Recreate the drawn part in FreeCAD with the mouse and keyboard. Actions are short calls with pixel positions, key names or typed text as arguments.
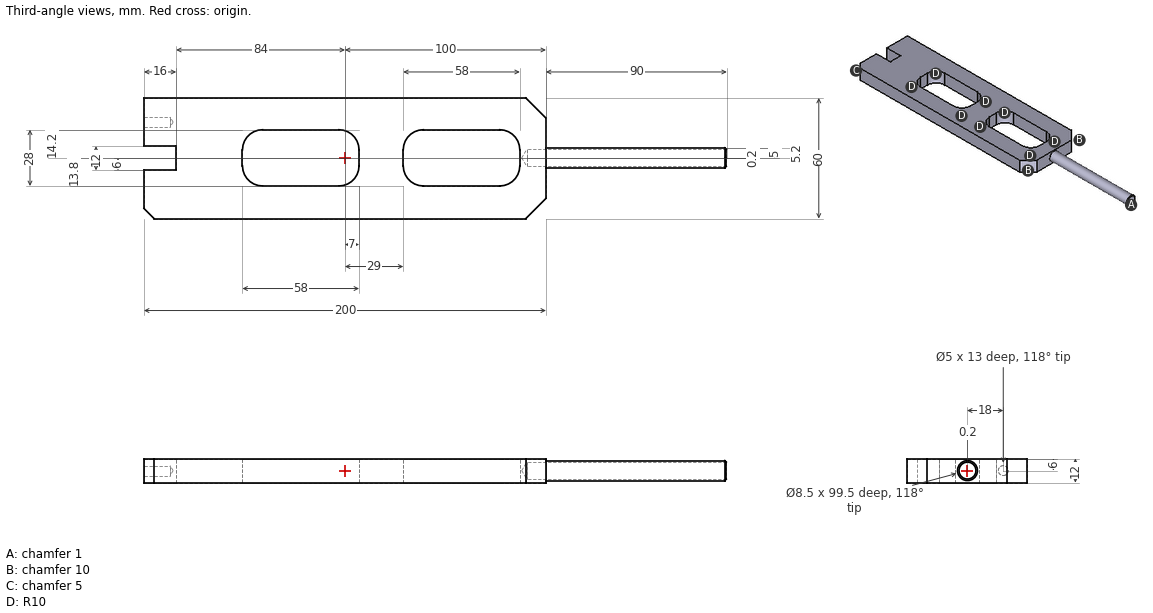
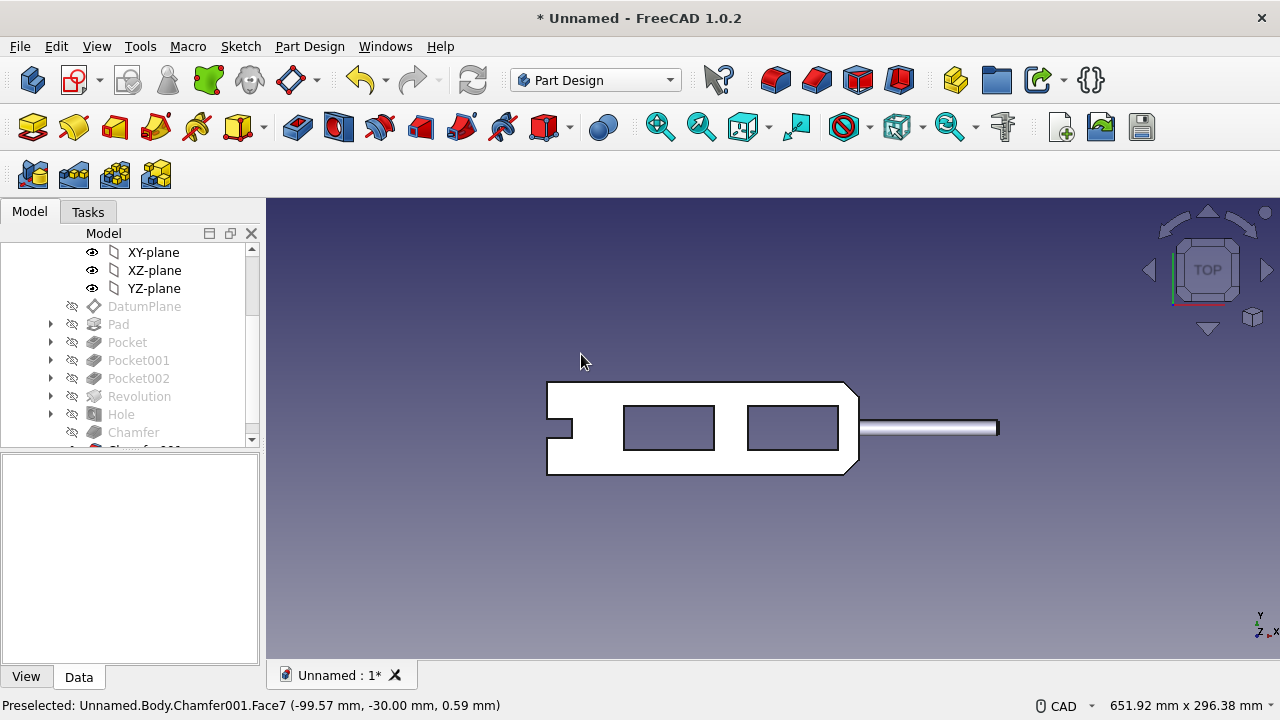
scroll(547, 474, up, 4)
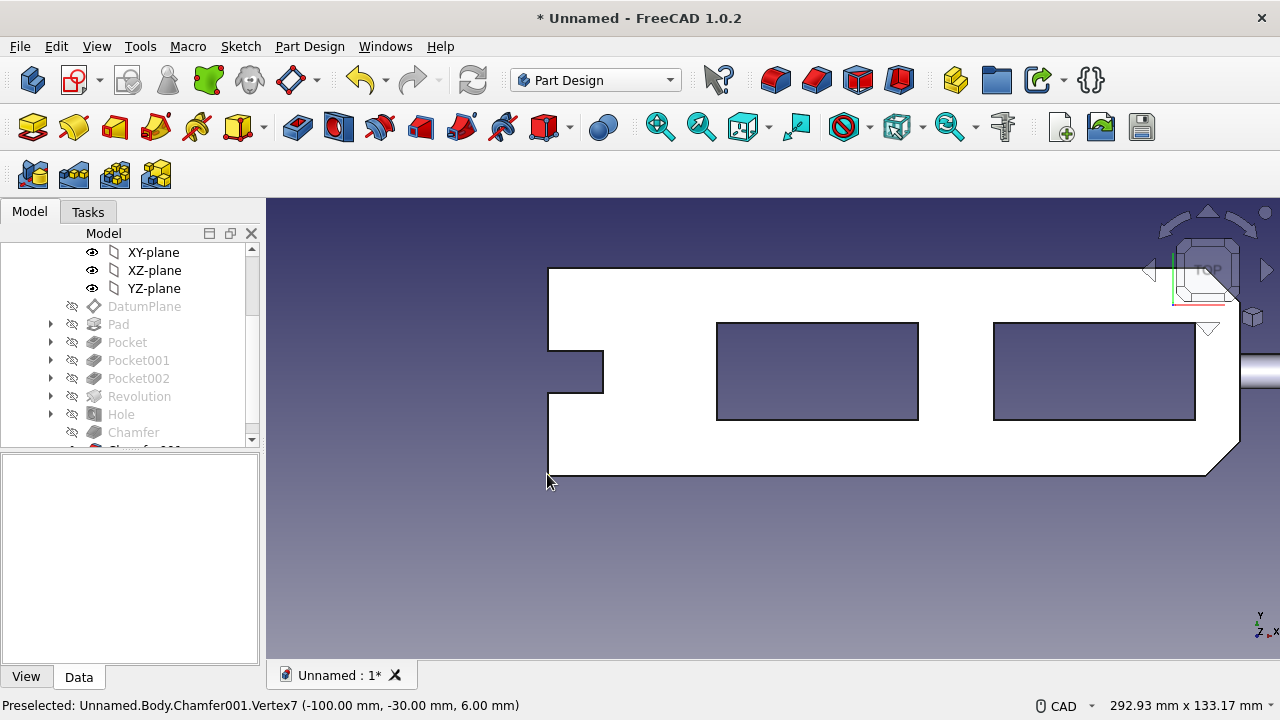
key(v)
key(f)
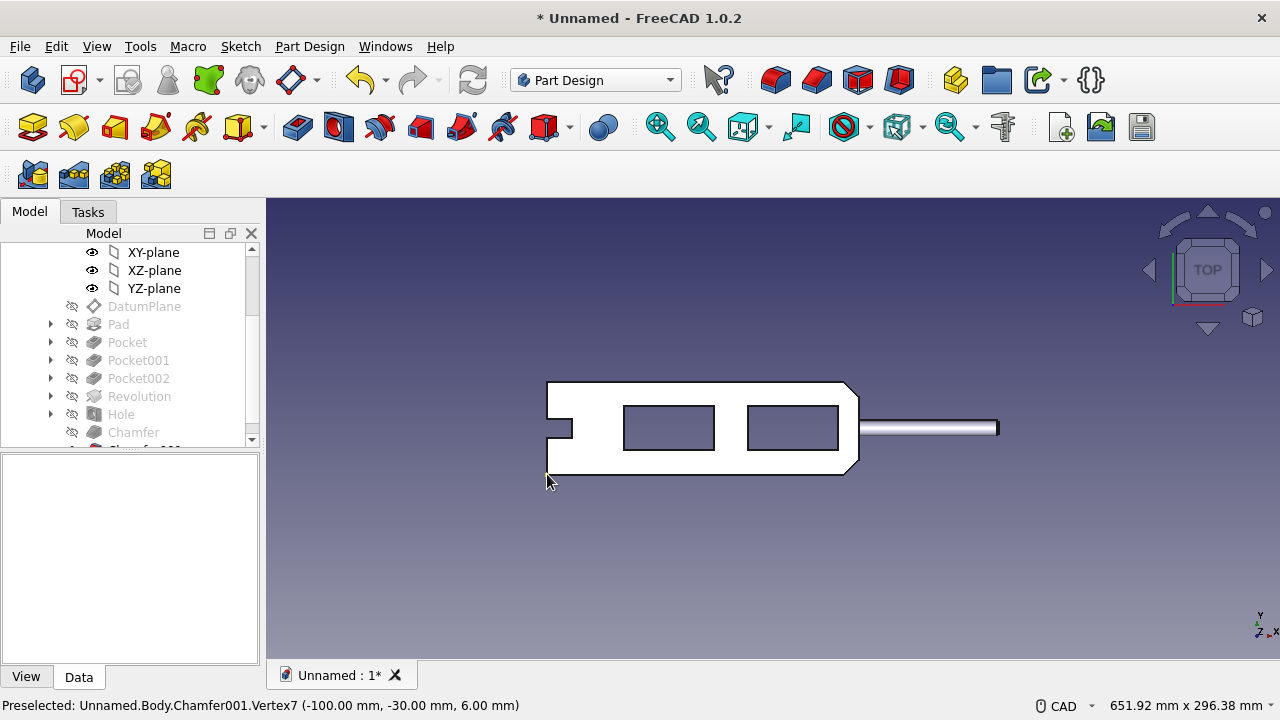
key(1)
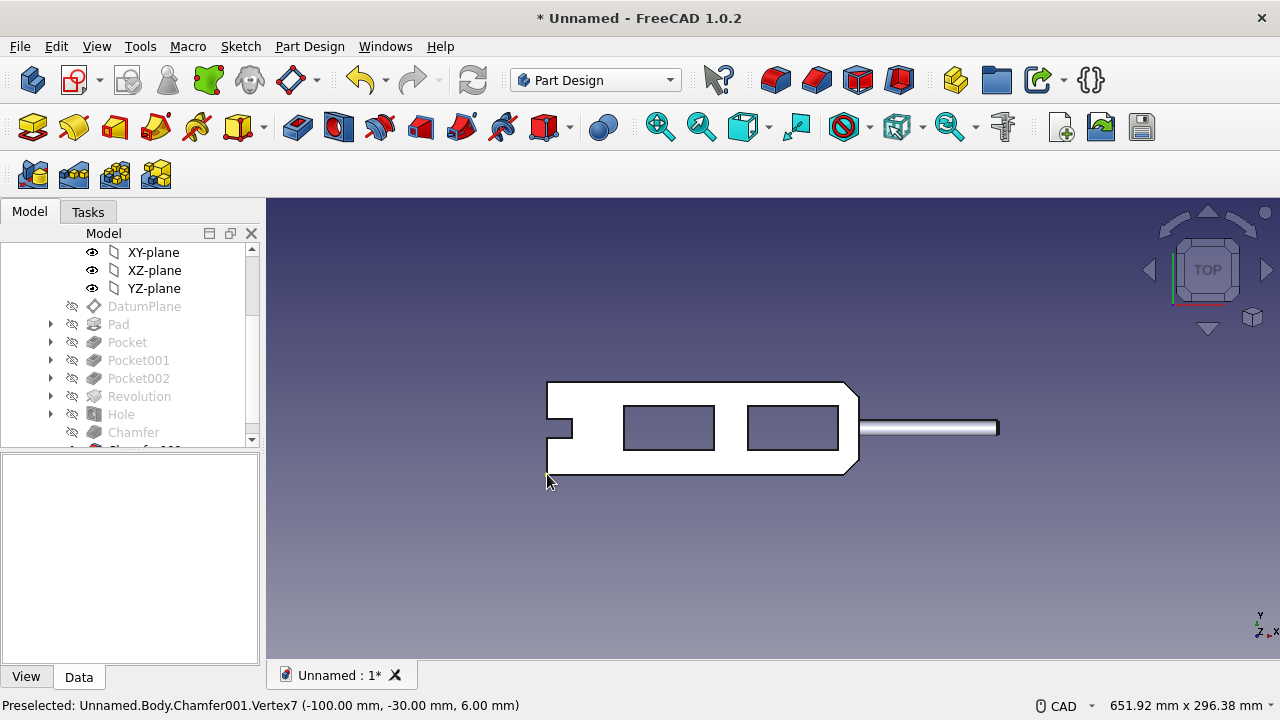
click(661, 128)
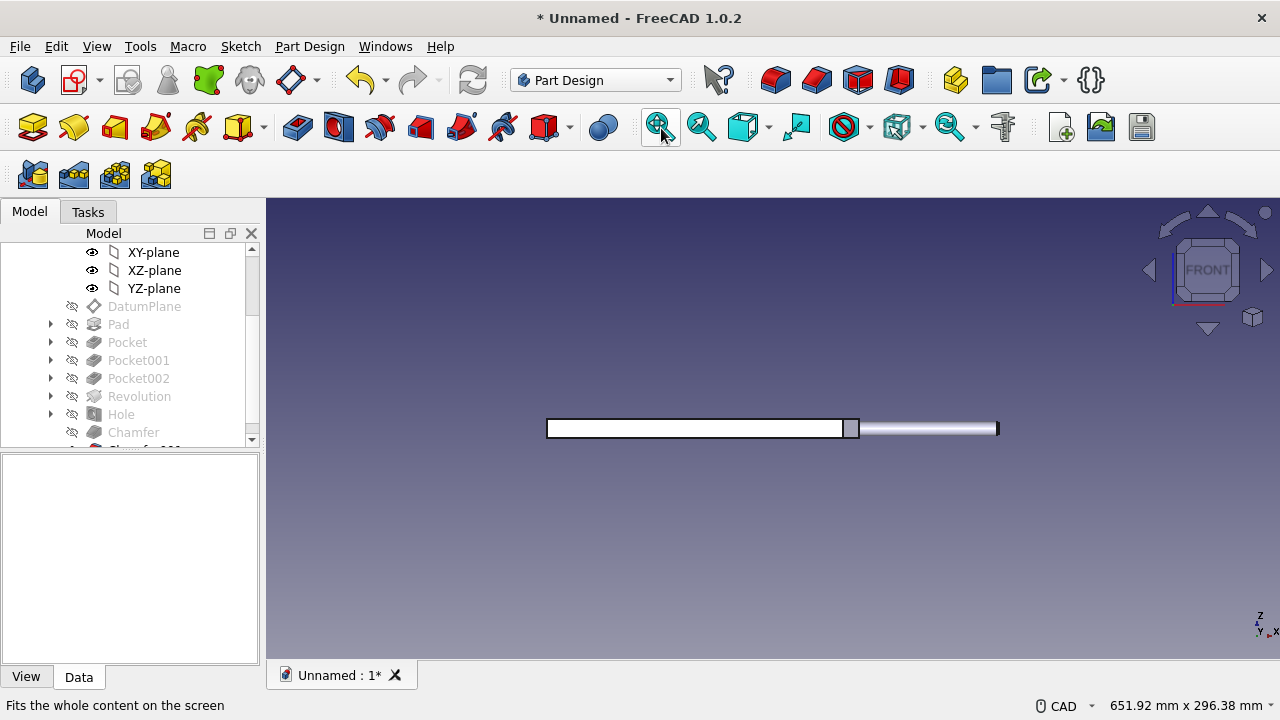
click(547, 428)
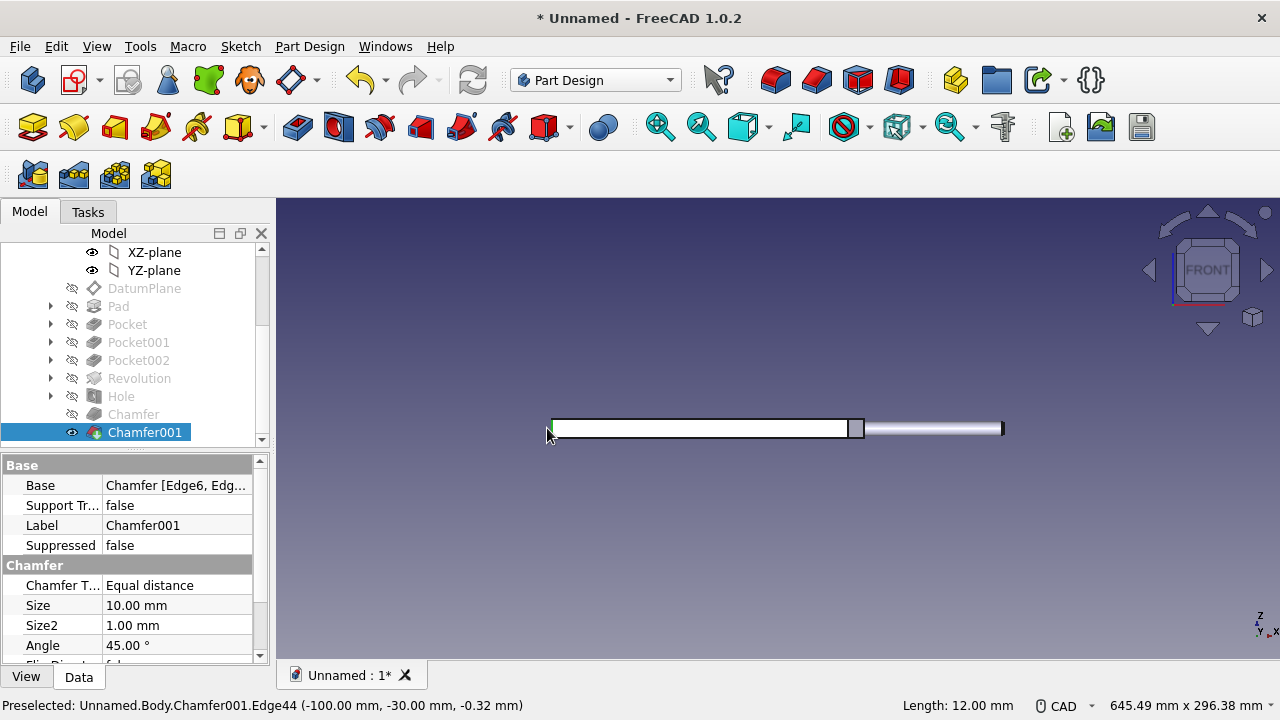
click(817, 80)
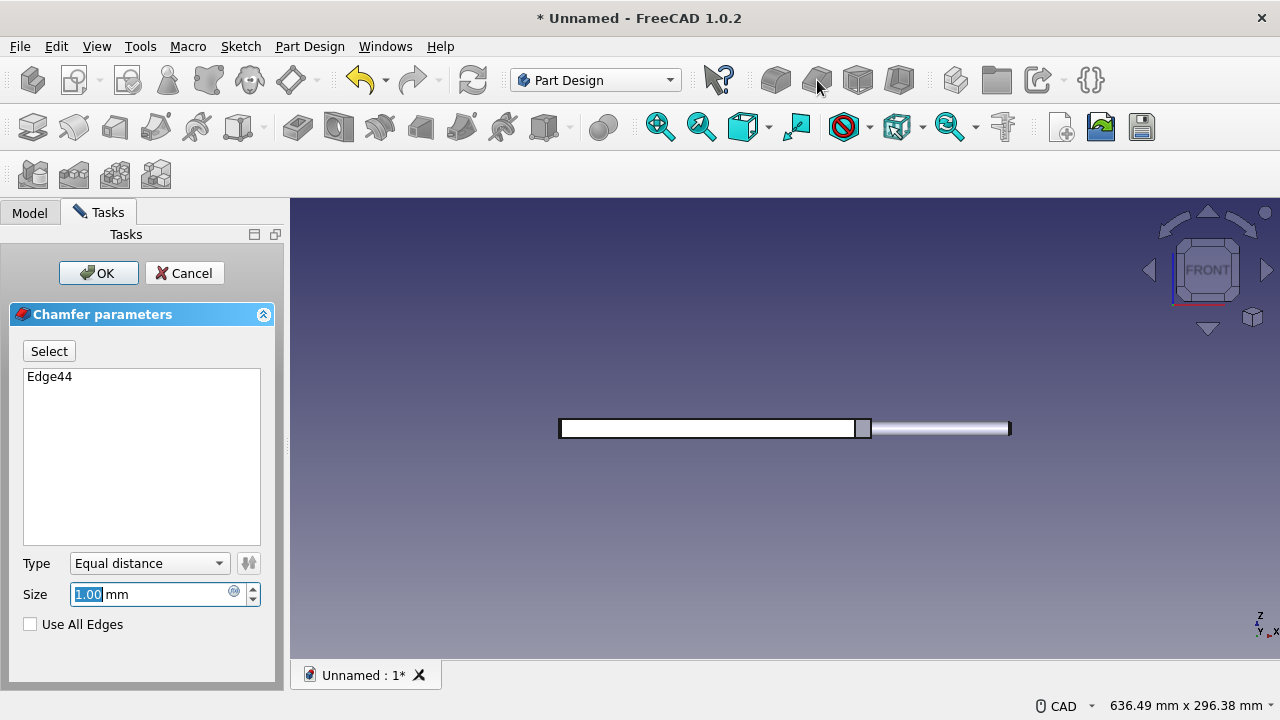
text(5)
key(Tab)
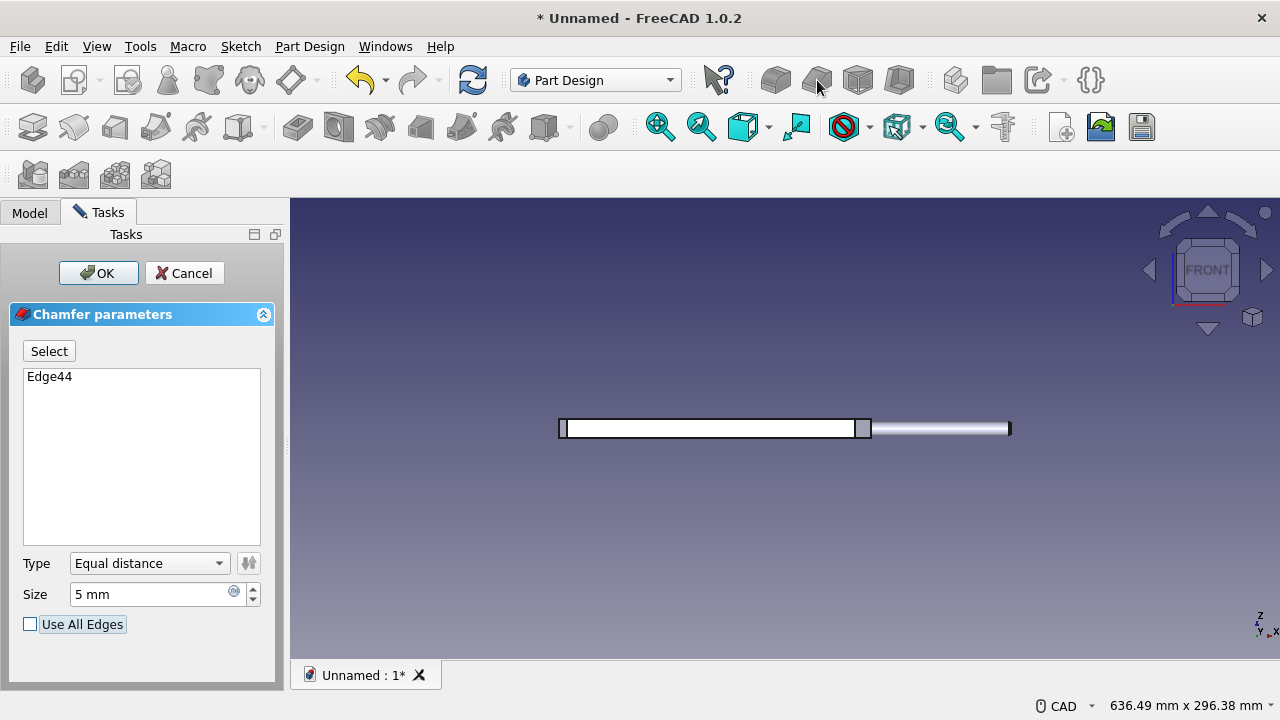
click(99, 273)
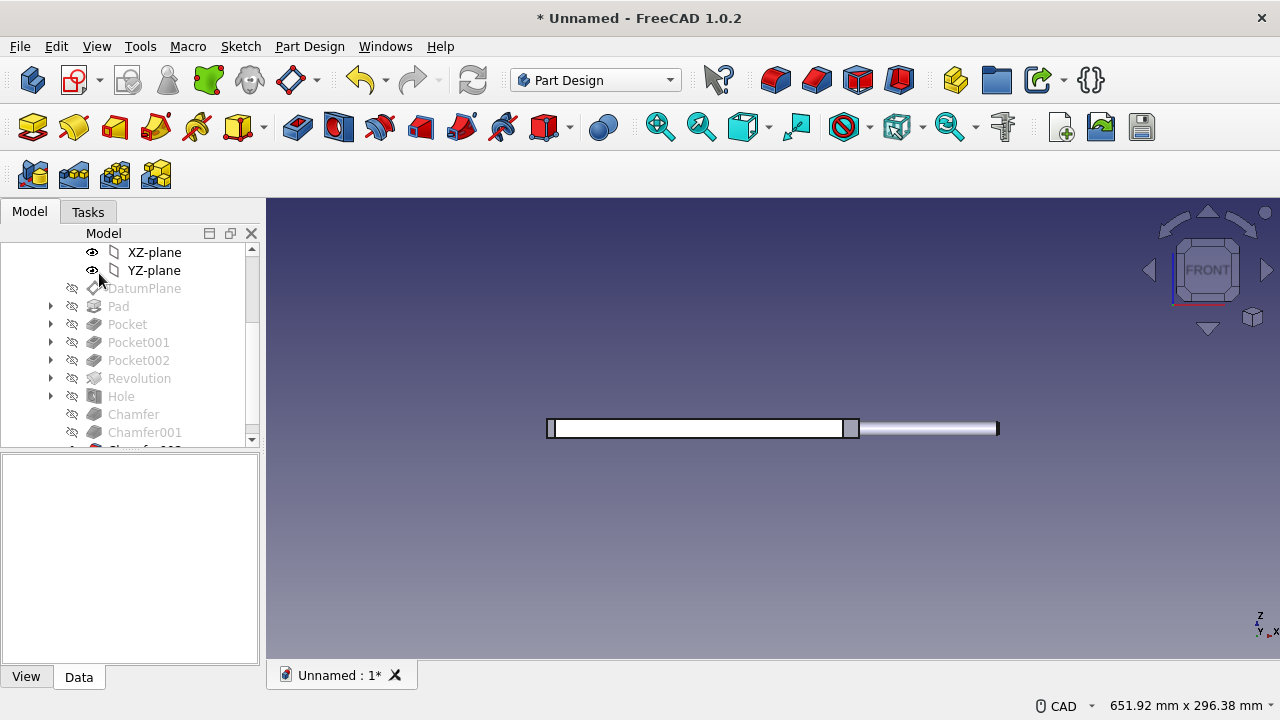
key(v)
key(f)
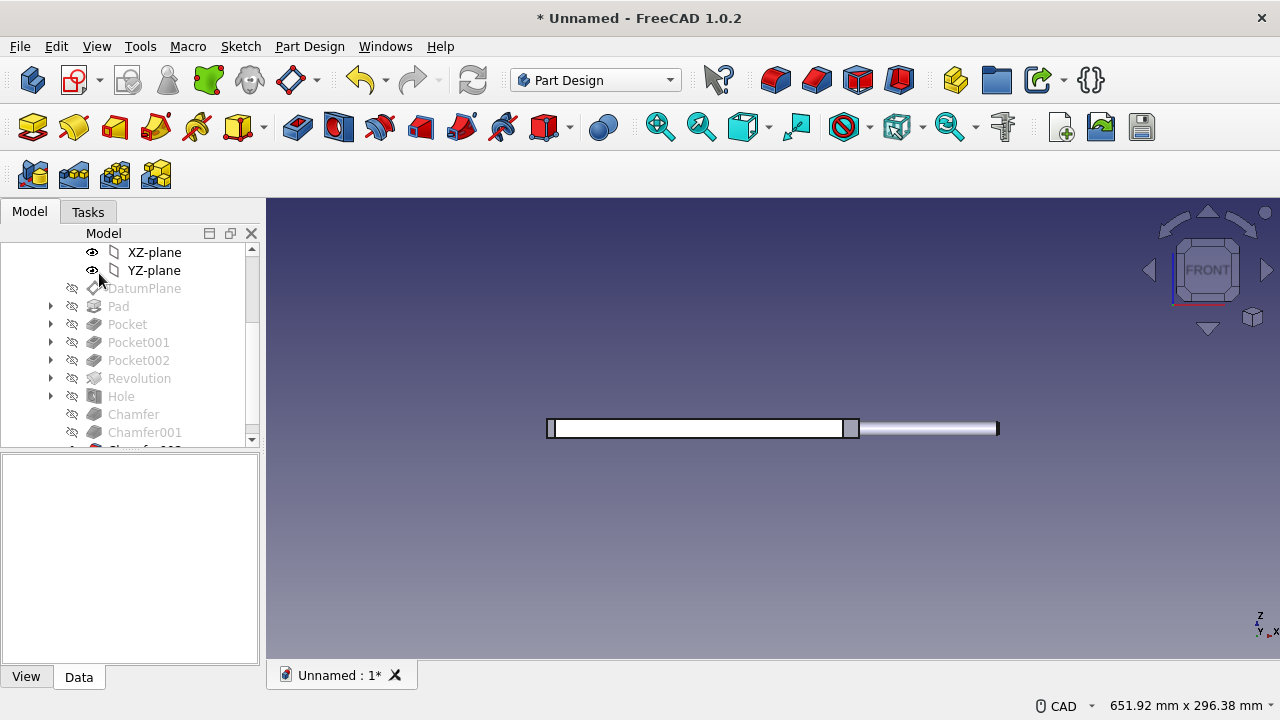
scroll(624, 428, up, 4)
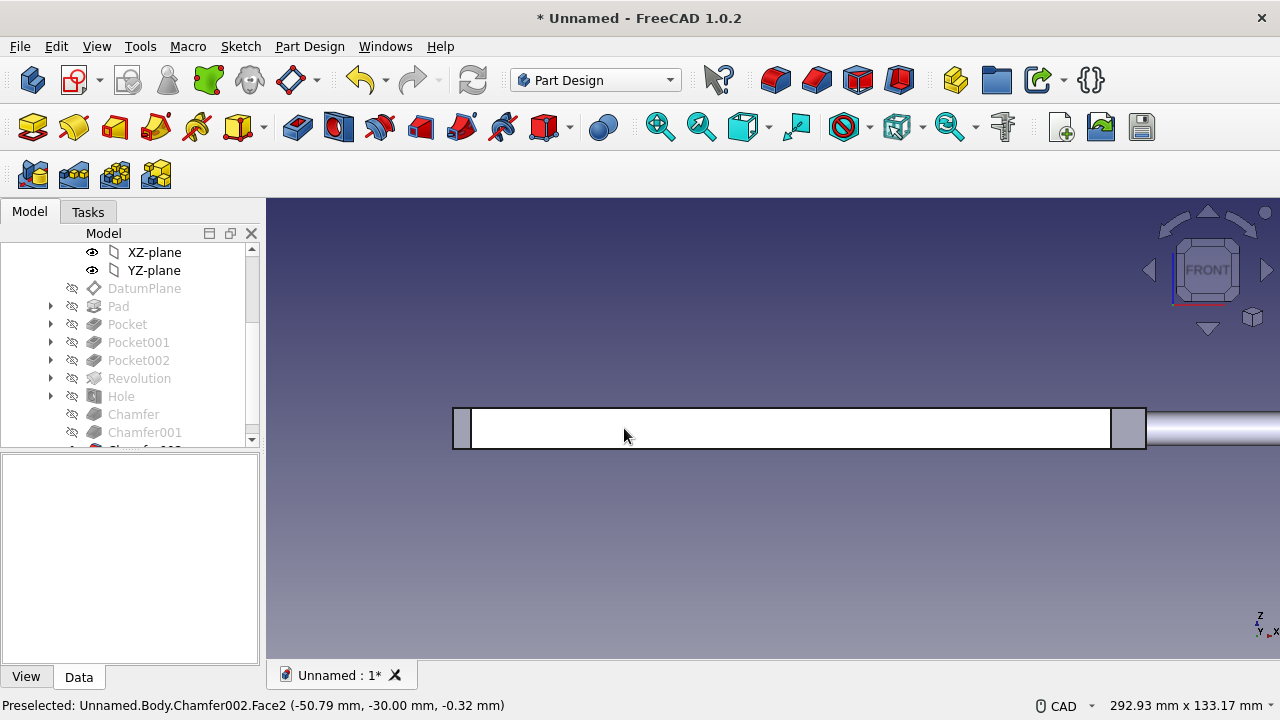
key(v)
key(f)